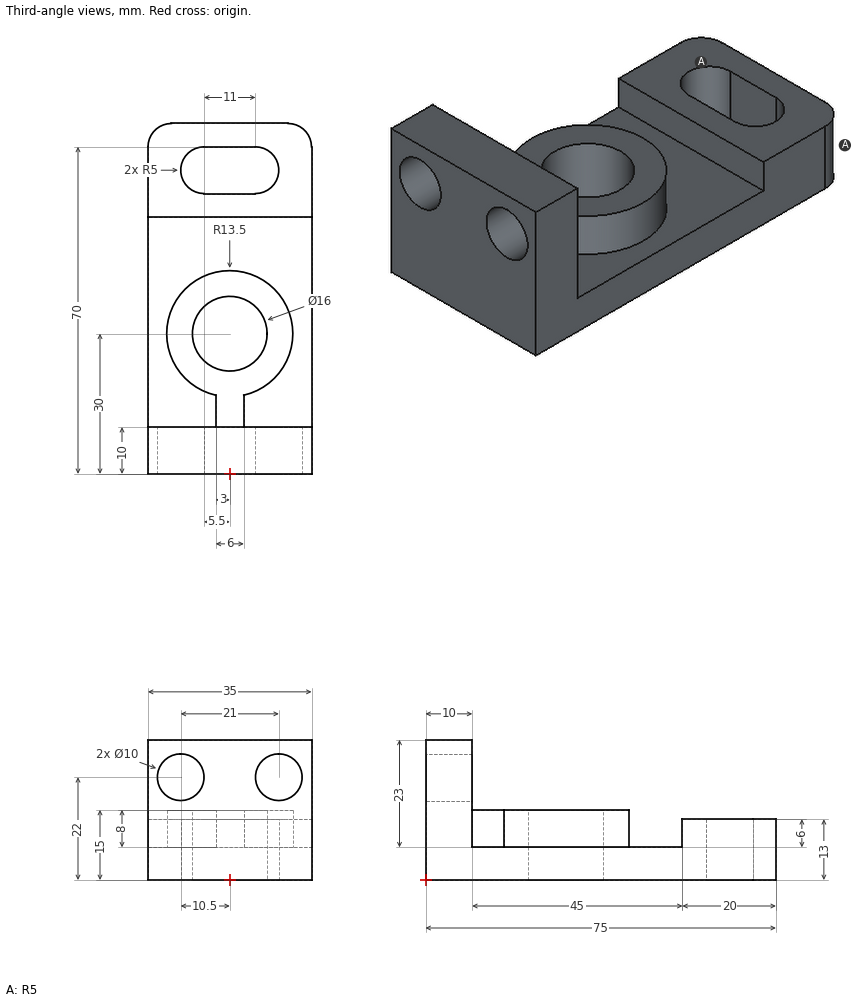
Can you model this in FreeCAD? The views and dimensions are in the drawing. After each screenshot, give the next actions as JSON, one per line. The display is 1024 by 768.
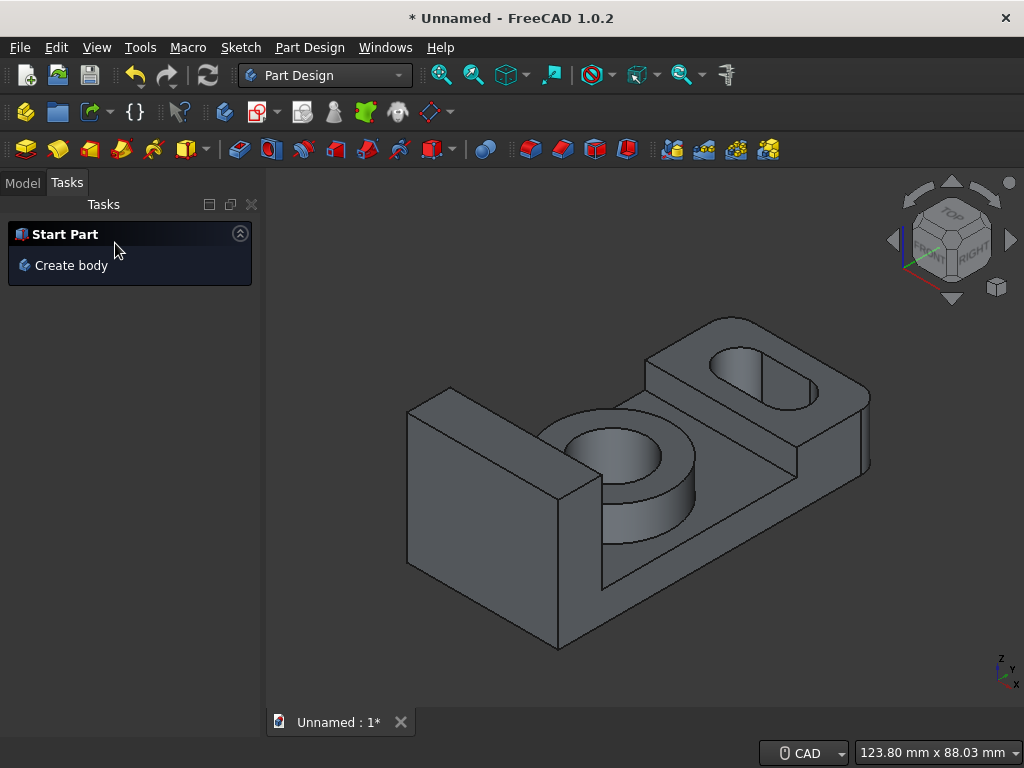
{"action": "key", "text": "4"}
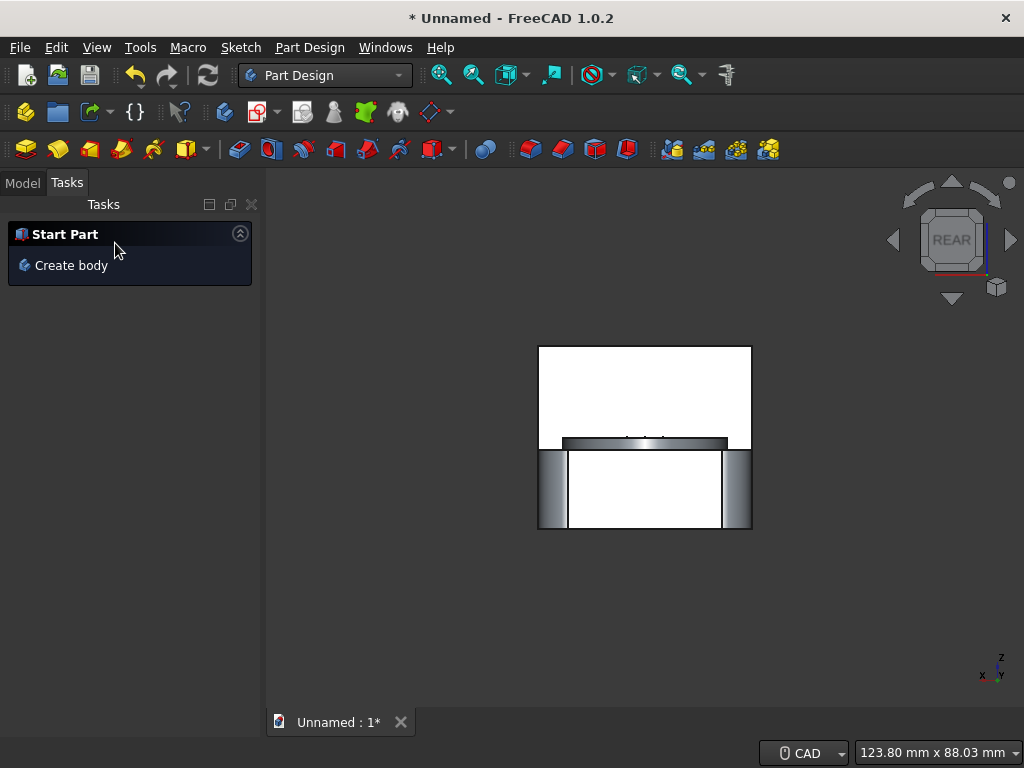
{"action": "key", "text": "v f"}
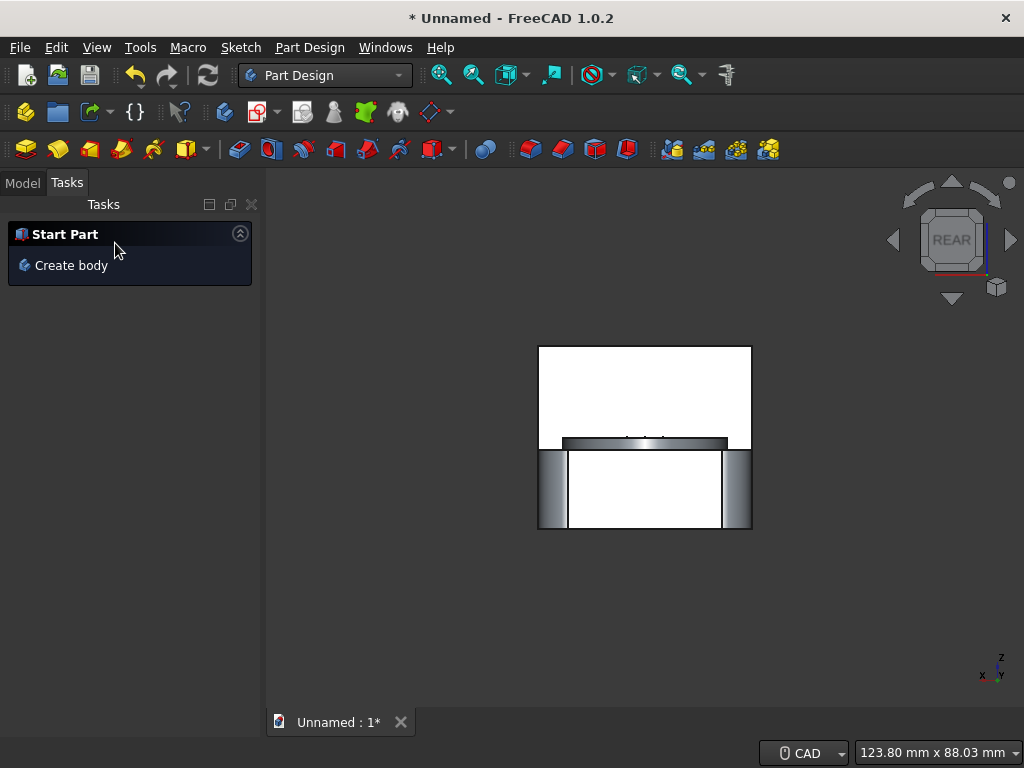
{"action": "left_click", "coordinate": [584, 415]}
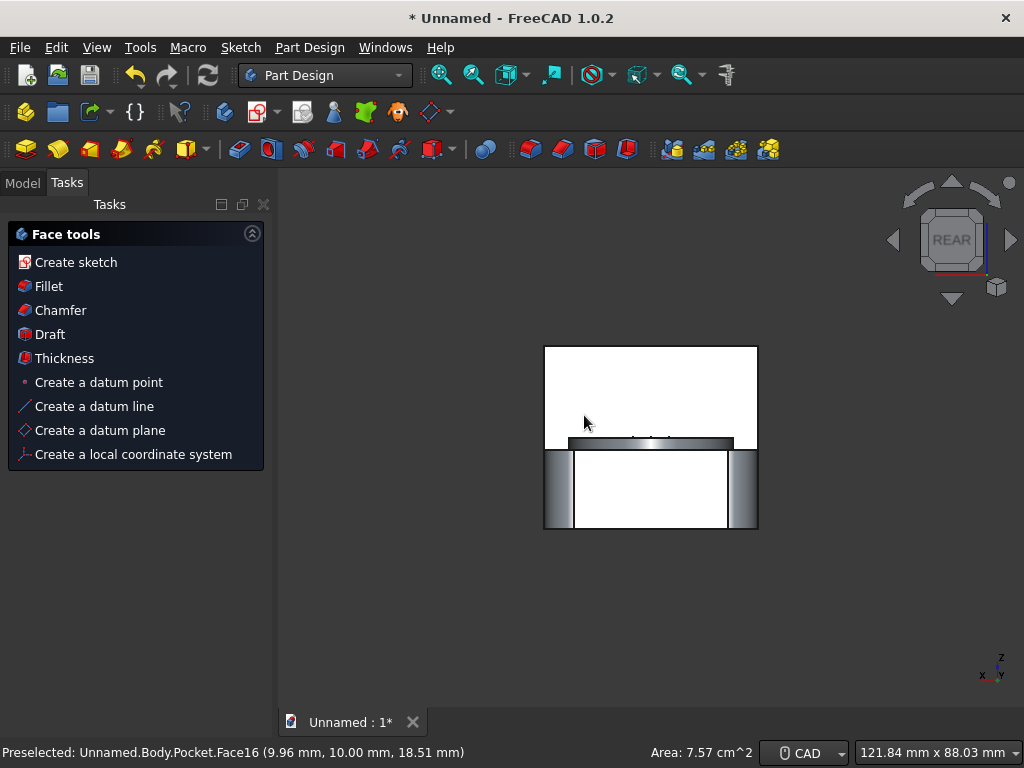
{"action": "left_click", "coordinate": [258, 112]}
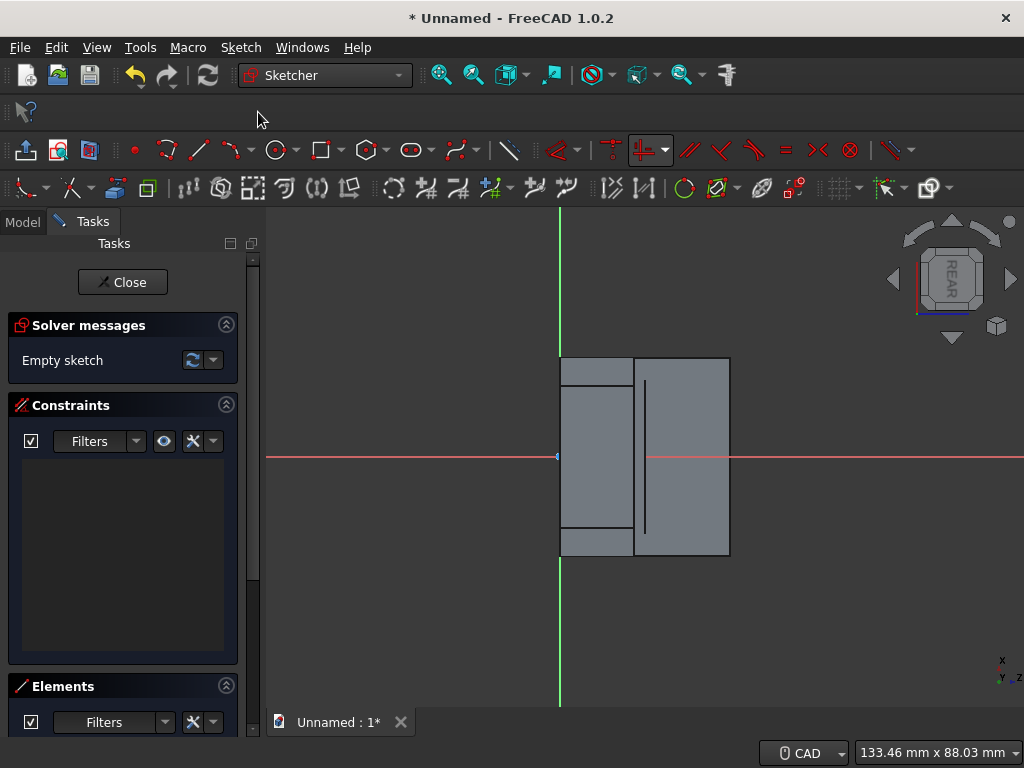
{"action": "scroll", "coordinate": [709, 457], "scroll_direction": "up", "scroll_amount": 3}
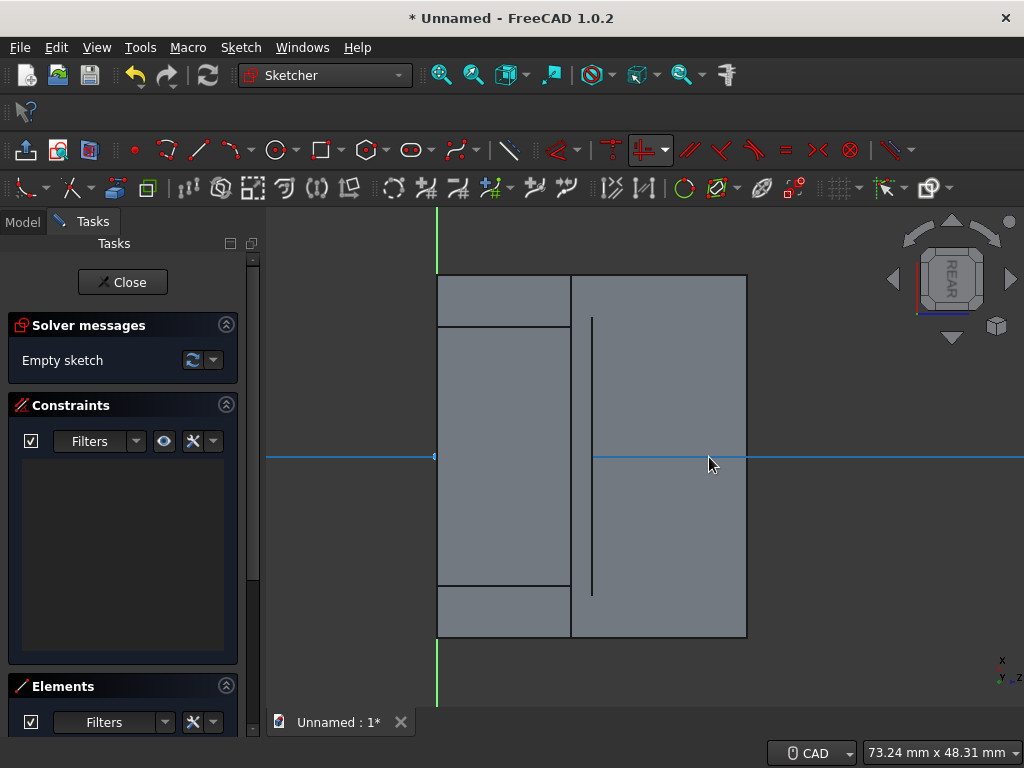
{"action": "key", "text": "g c"}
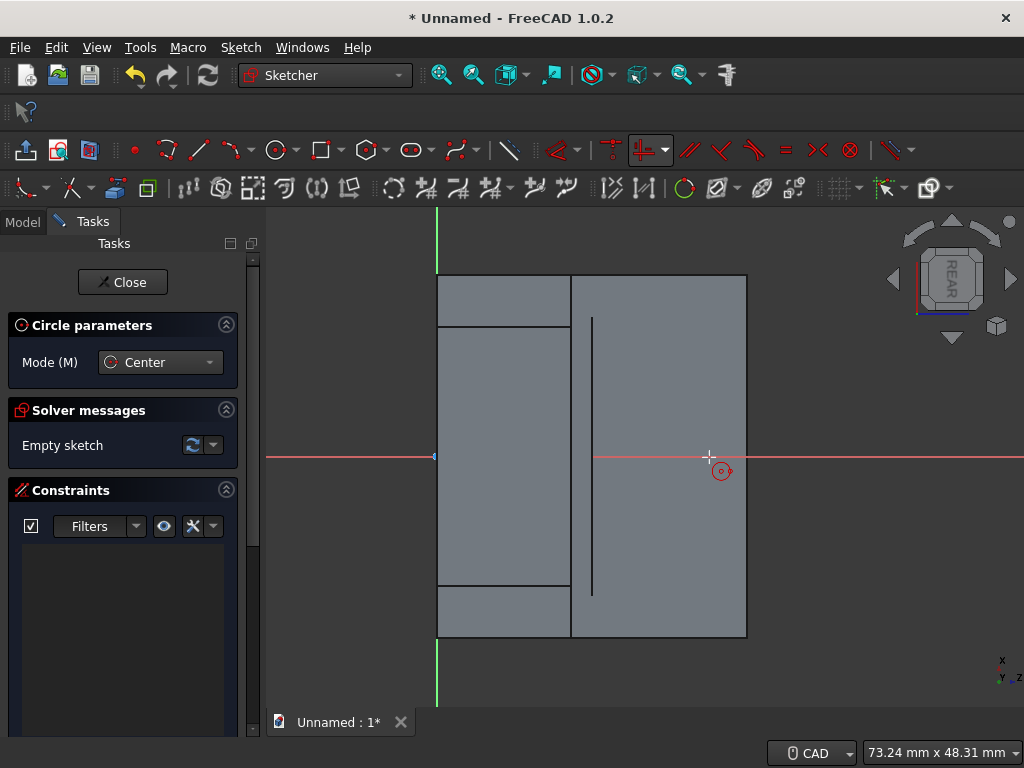
{"action": "left_click", "coordinate": [664, 565]}
{"action": "mouse_move", "coordinate": [701, 529]}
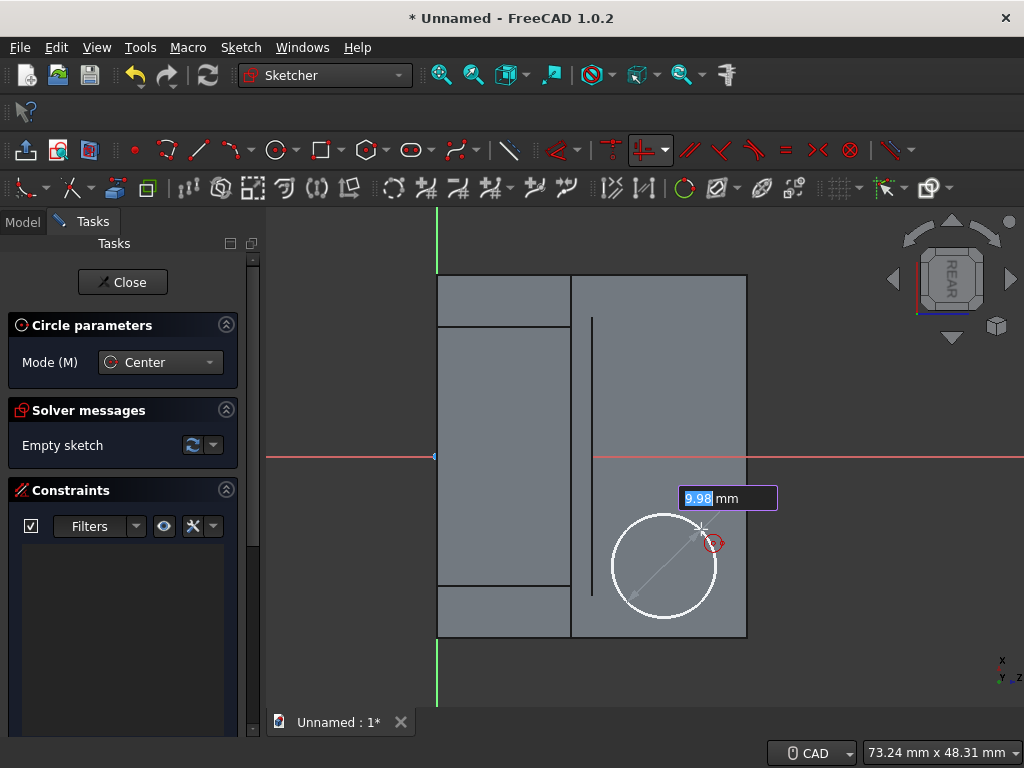
{"action": "type", "text": "10"}
{"action": "key", "text": "Return"}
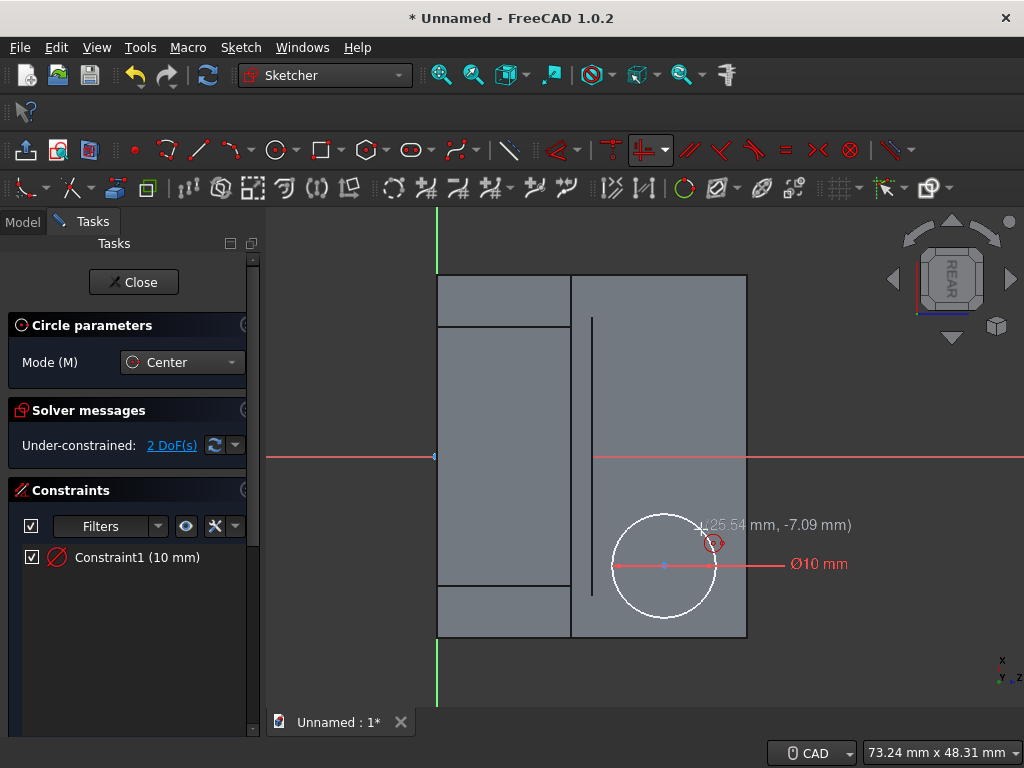
{"action": "left_click", "coordinate": [664, 348]}
{"action": "mouse_move", "coordinate": [701, 311]}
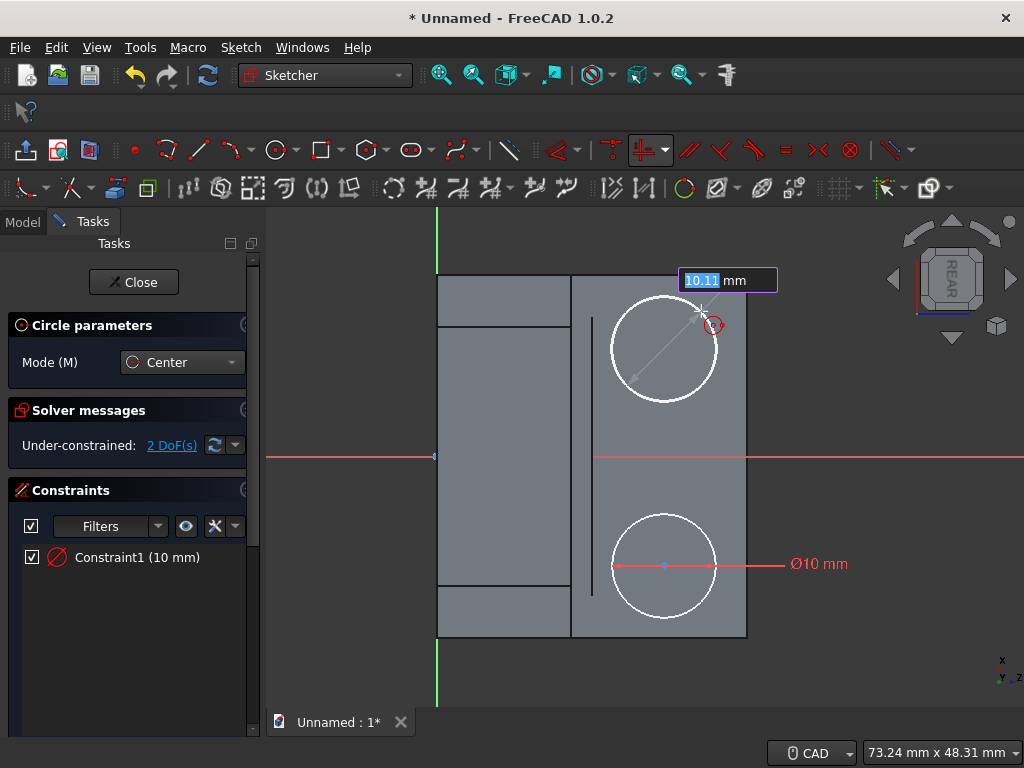
{"action": "type", "text": "10"}
{"action": "key", "text": "Return"}
{"action": "key", "text": "Escape"}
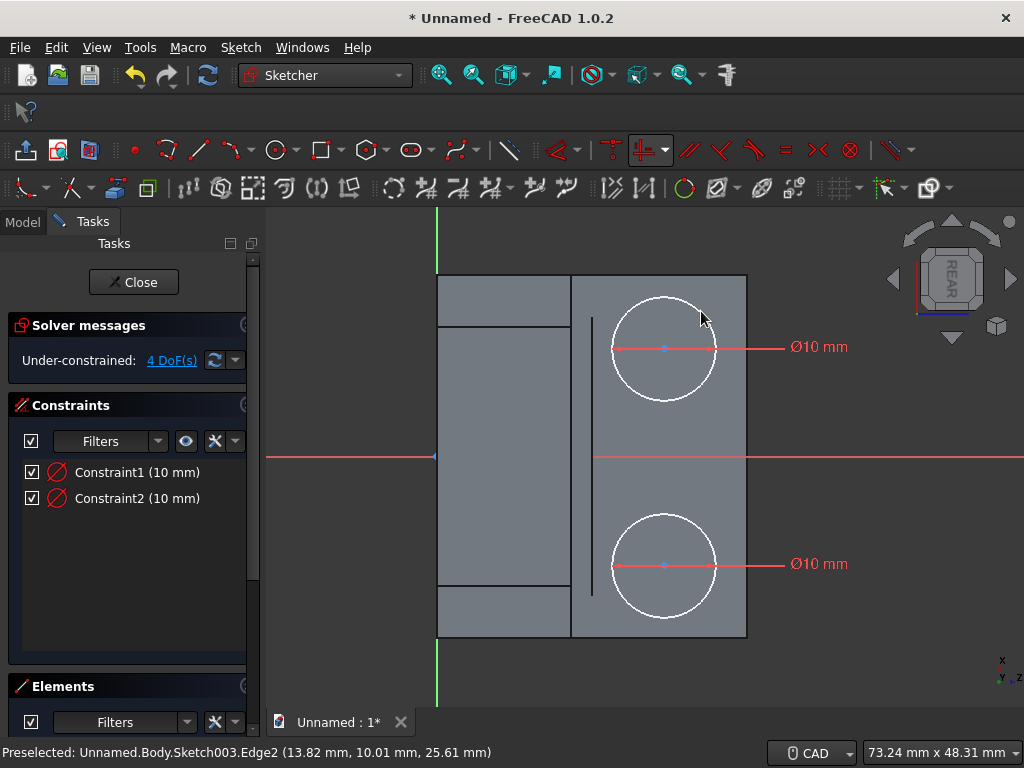
{"action": "left_click", "coordinate": [664, 566]}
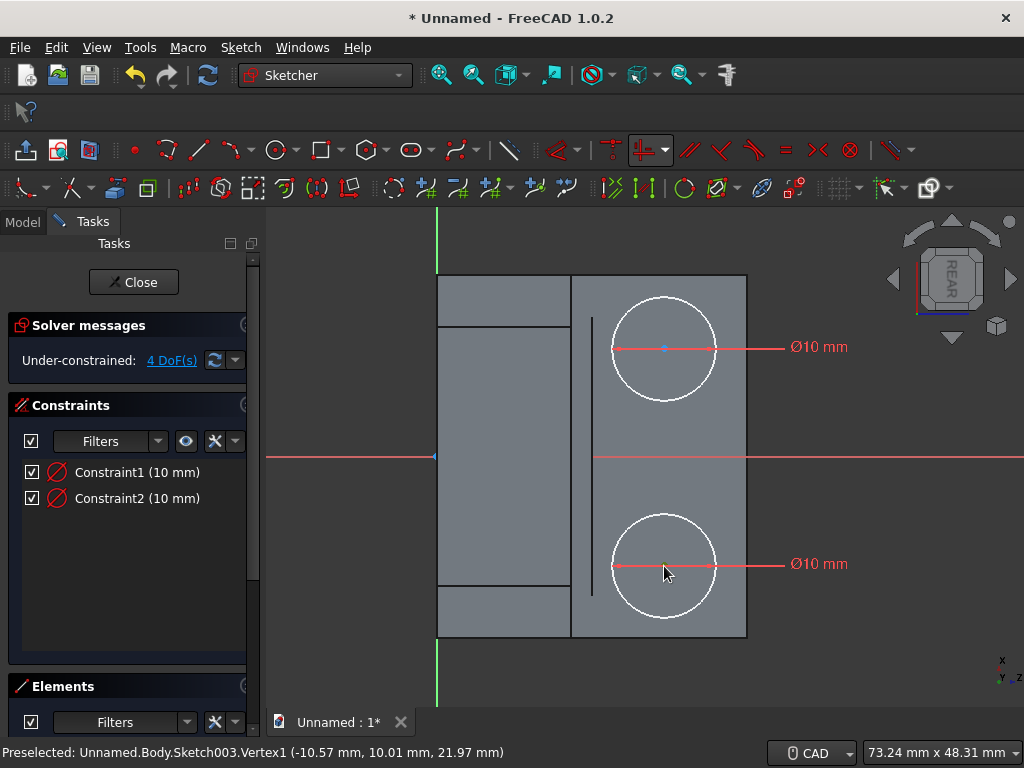
{"action": "left_click", "coordinate": [664, 349]}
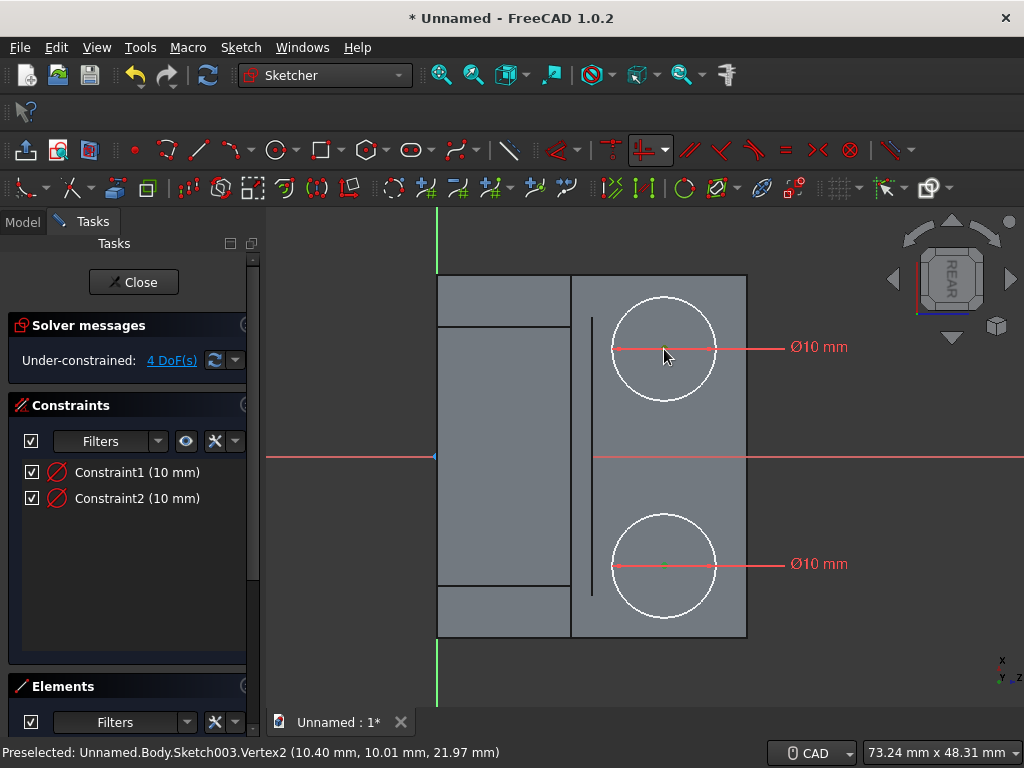
{"action": "key", "text": "v"}